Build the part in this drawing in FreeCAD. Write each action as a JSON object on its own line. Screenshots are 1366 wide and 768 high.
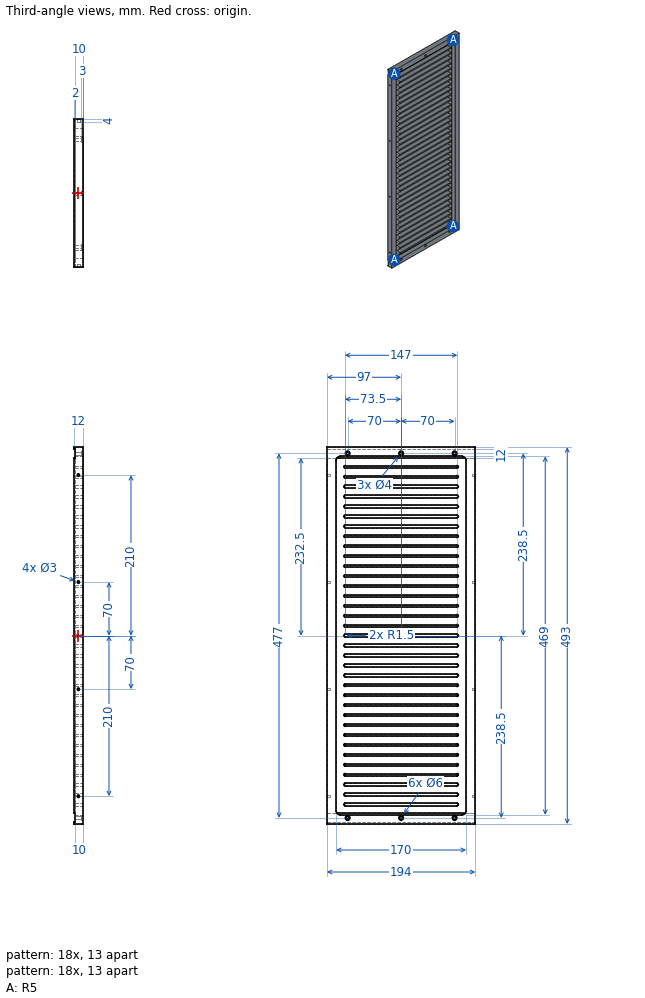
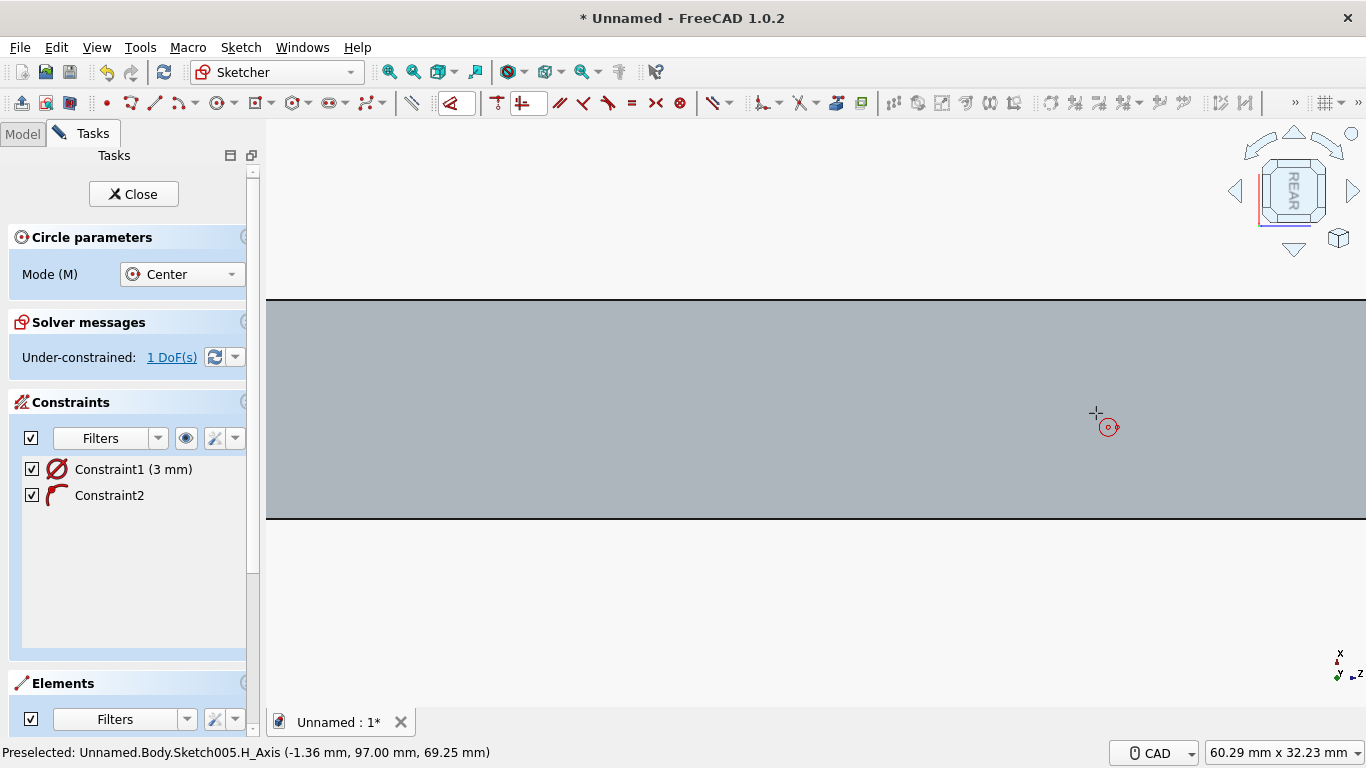
{"action": "scroll", "coordinate": [1096, 413], "scroll_direction": "down", "scroll_amount": 12}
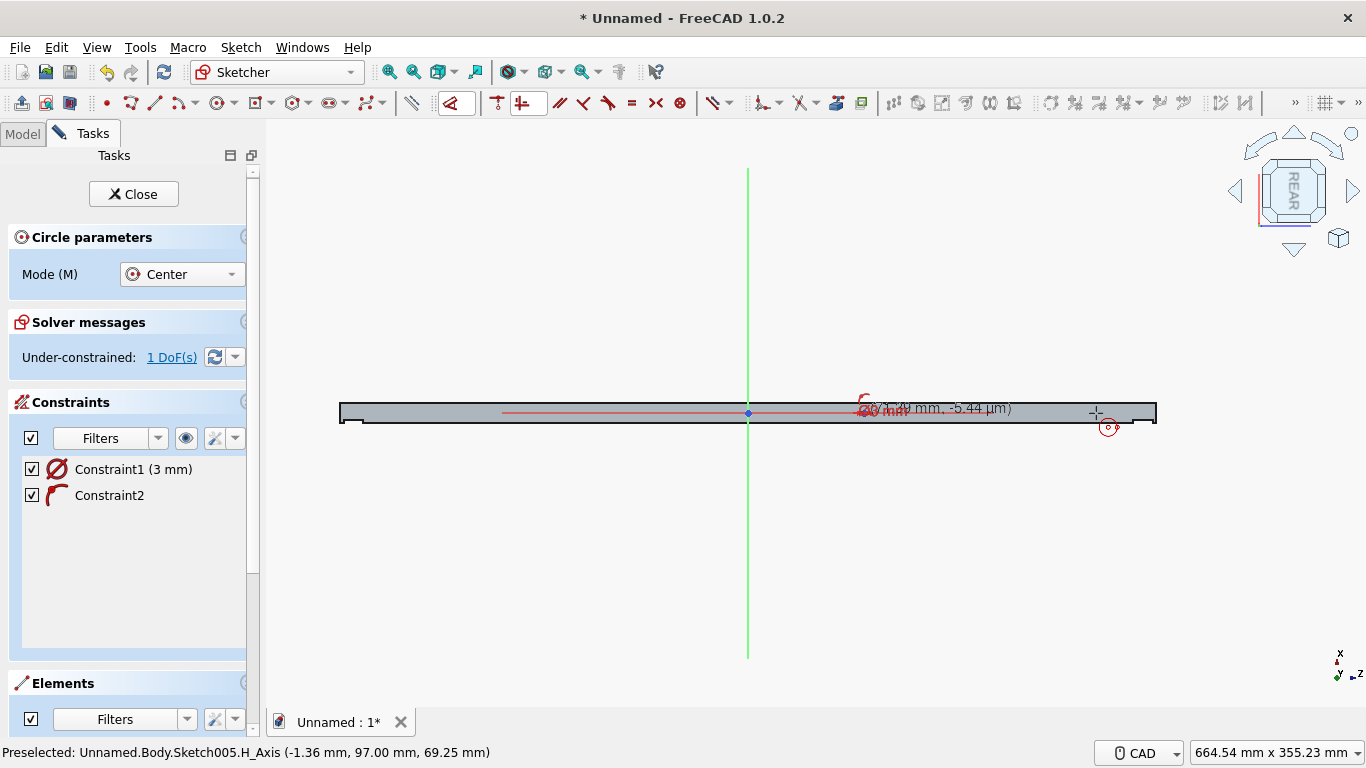
{"action": "left_click", "coordinate": [1096, 413]}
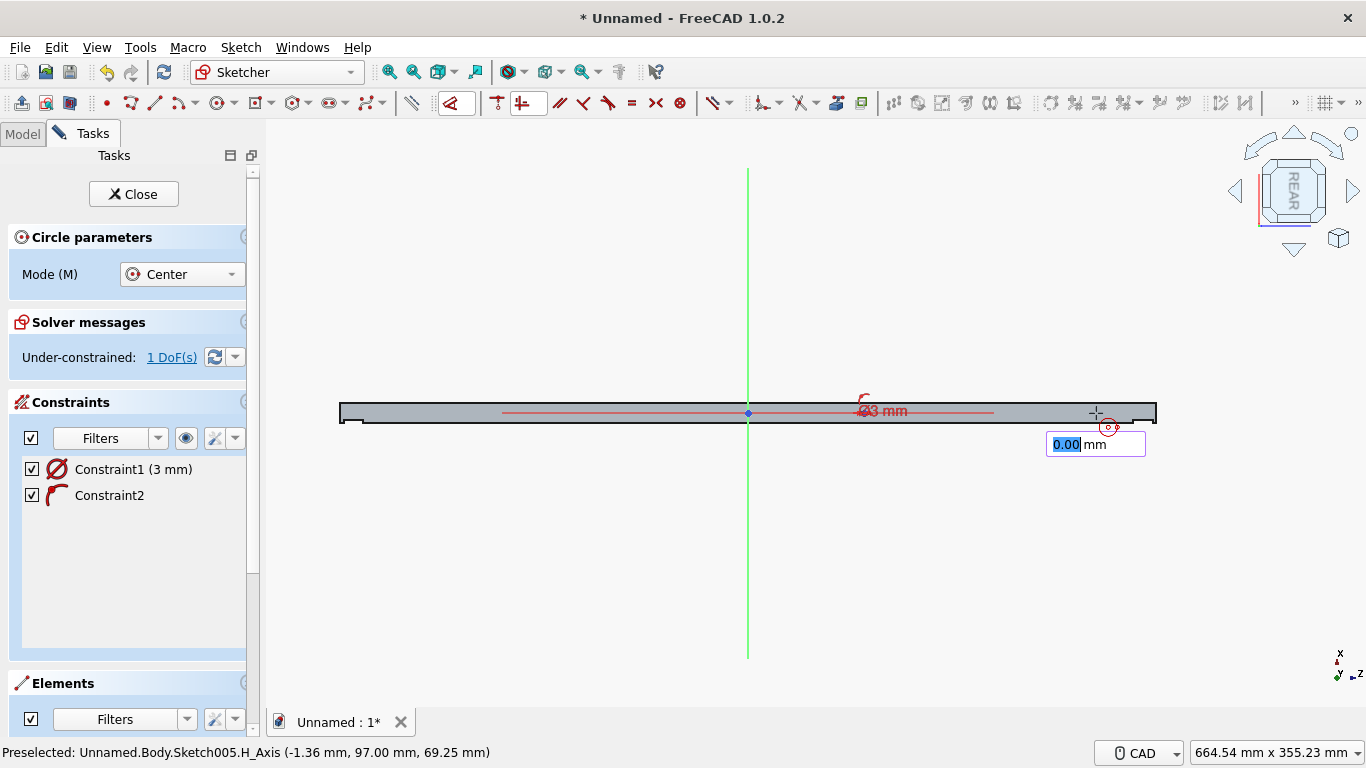
{"action": "scroll", "coordinate": [1095, 415], "scroll_direction": "up", "scroll_amount": 10}
{"action": "mouse_move", "coordinate": [1091, 415]}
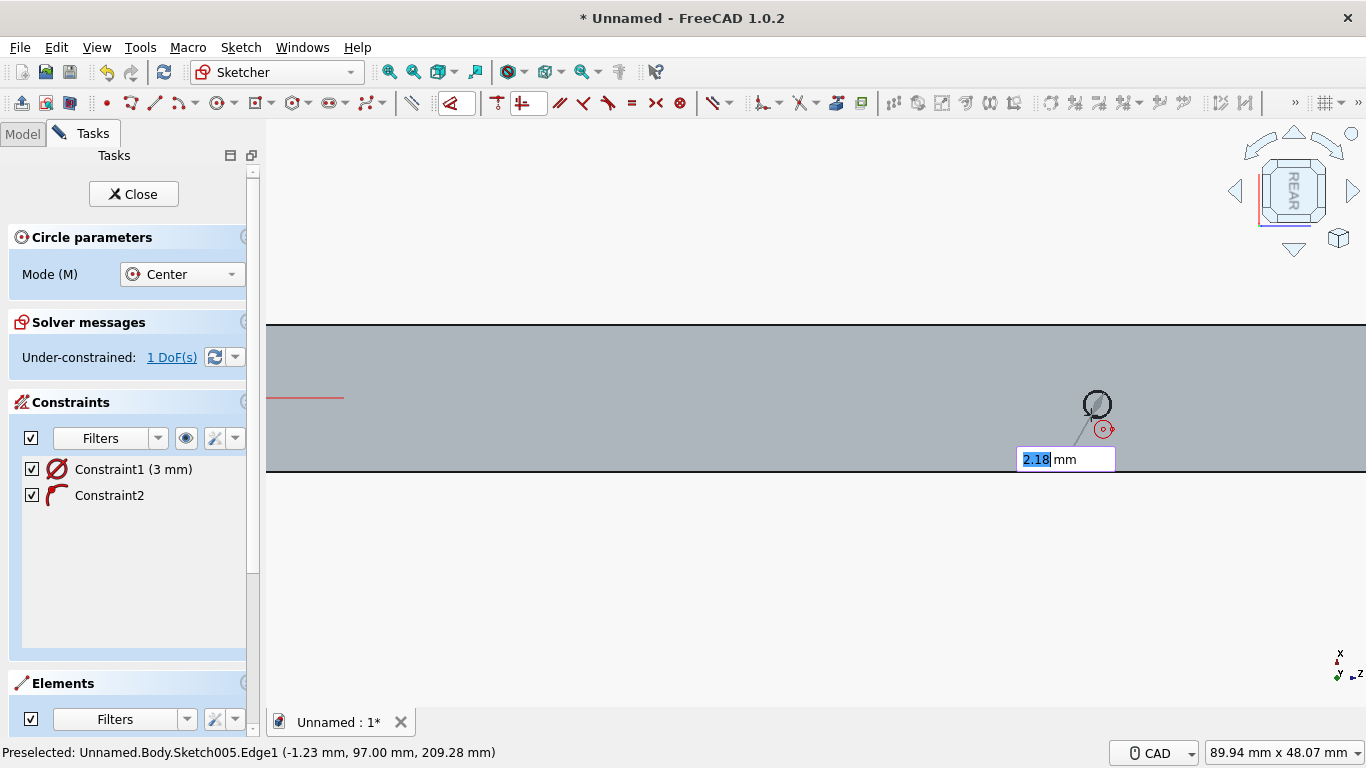
{"action": "type", "text": "3"}
{"action": "key", "text": "Return"}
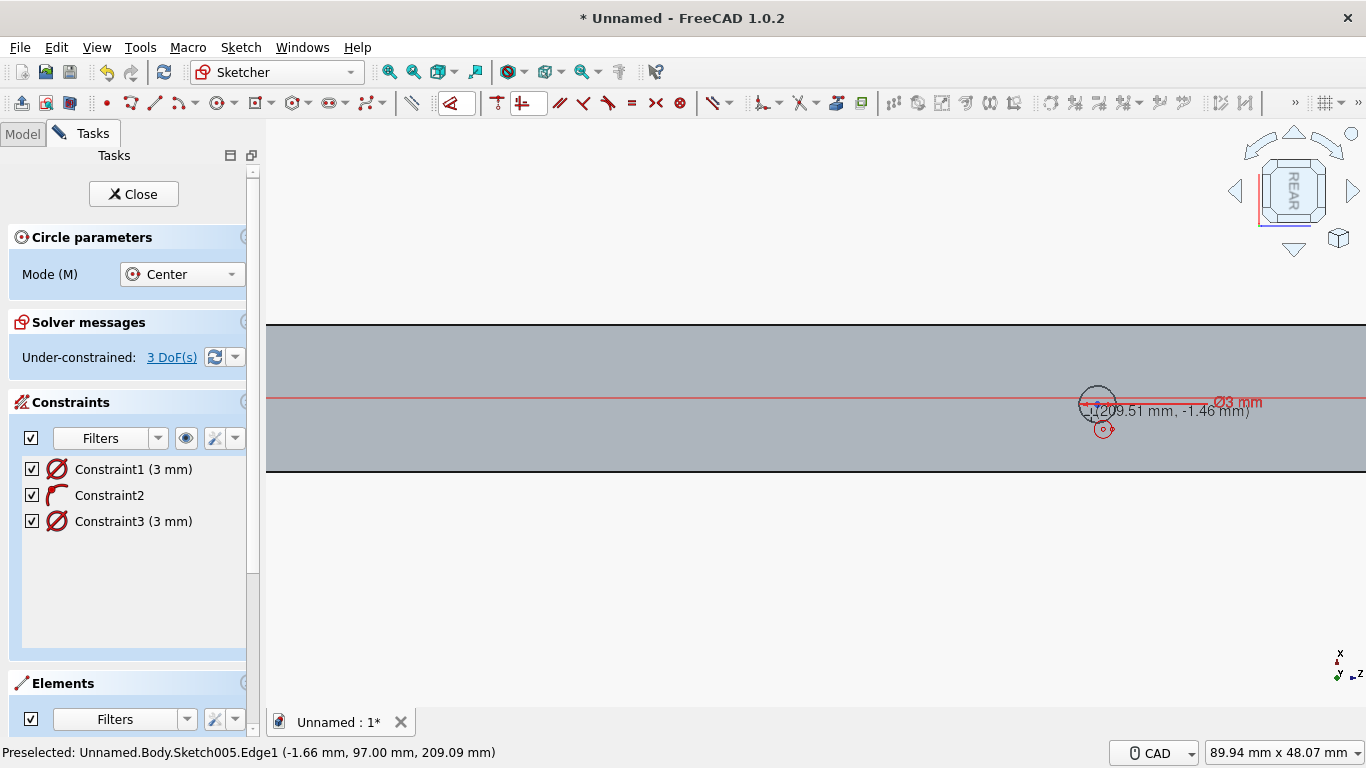
{"action": "scroll", "coordinate": [1095, 415], "scroll_direction": "down", "scroll_amount": 10}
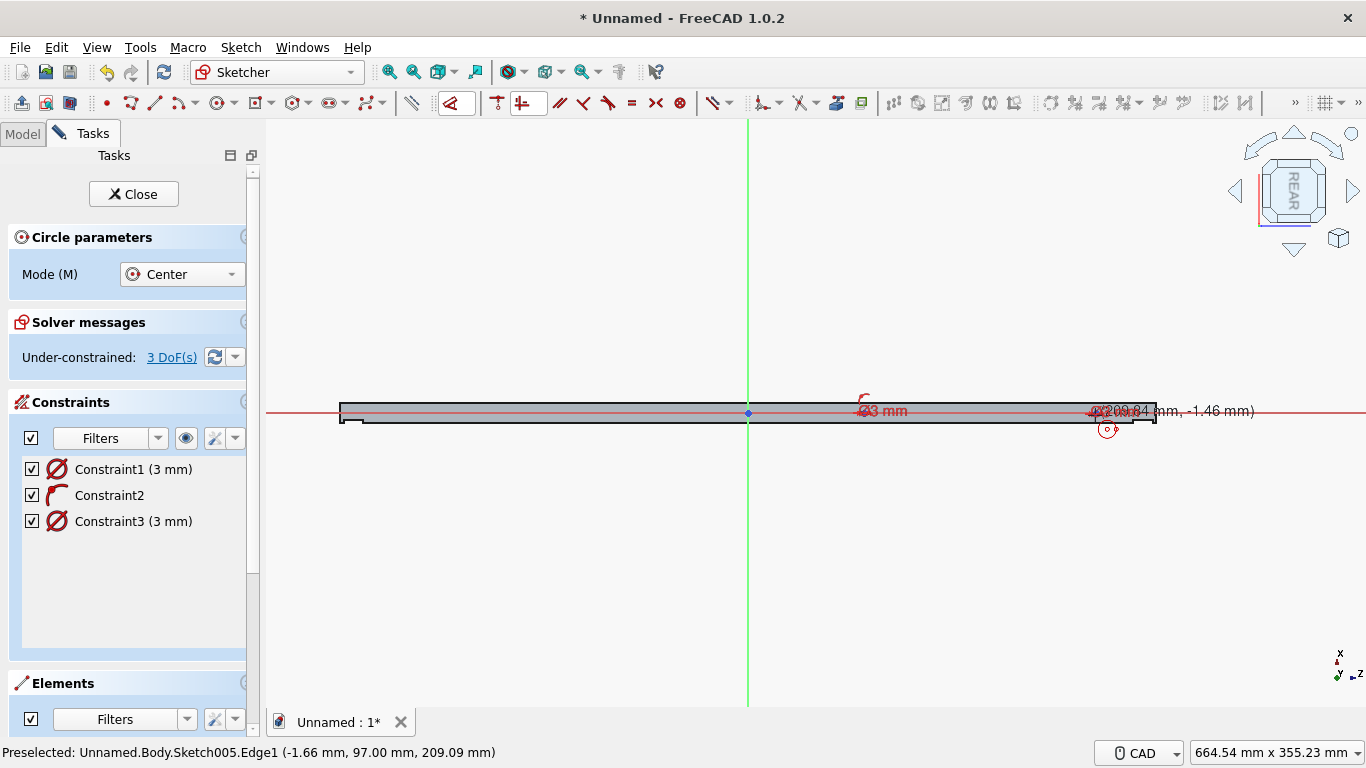
{"action": "scroll", "coordinate": [401, 413], "scroll_direction": "up", "scroll_amount": 12}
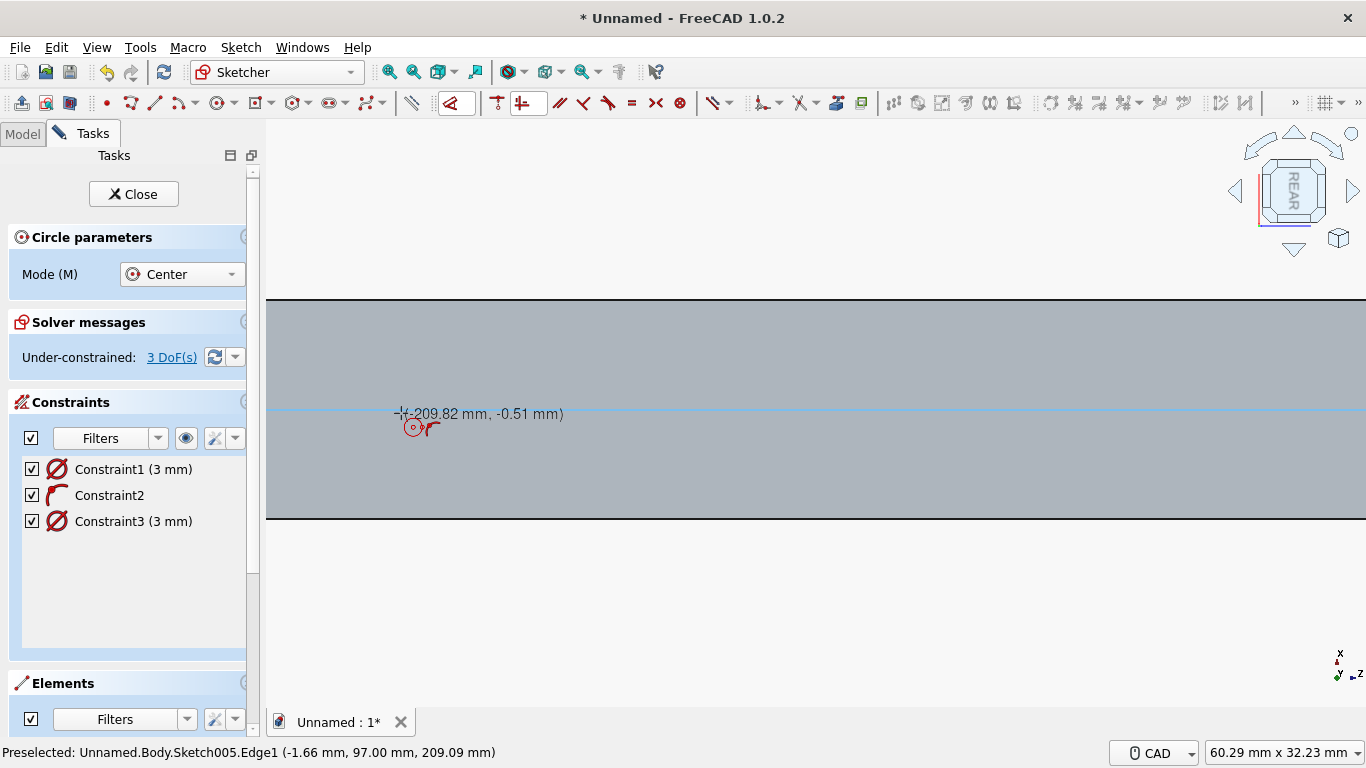
{"action": "scroll", "coordinate": [400, 413], "scroll_direction": "down", "scroll_amount": 12}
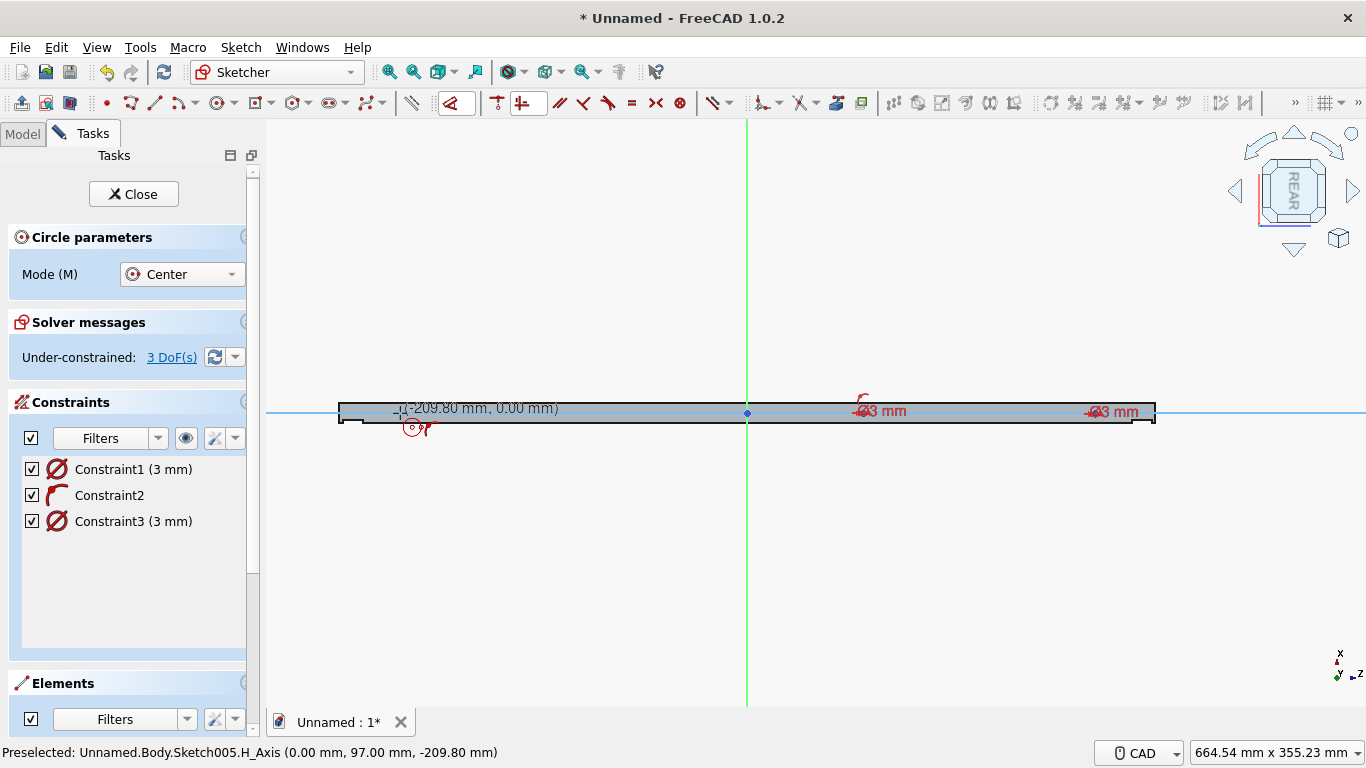
{"action": "left_click", "coordinate": [400, 413]}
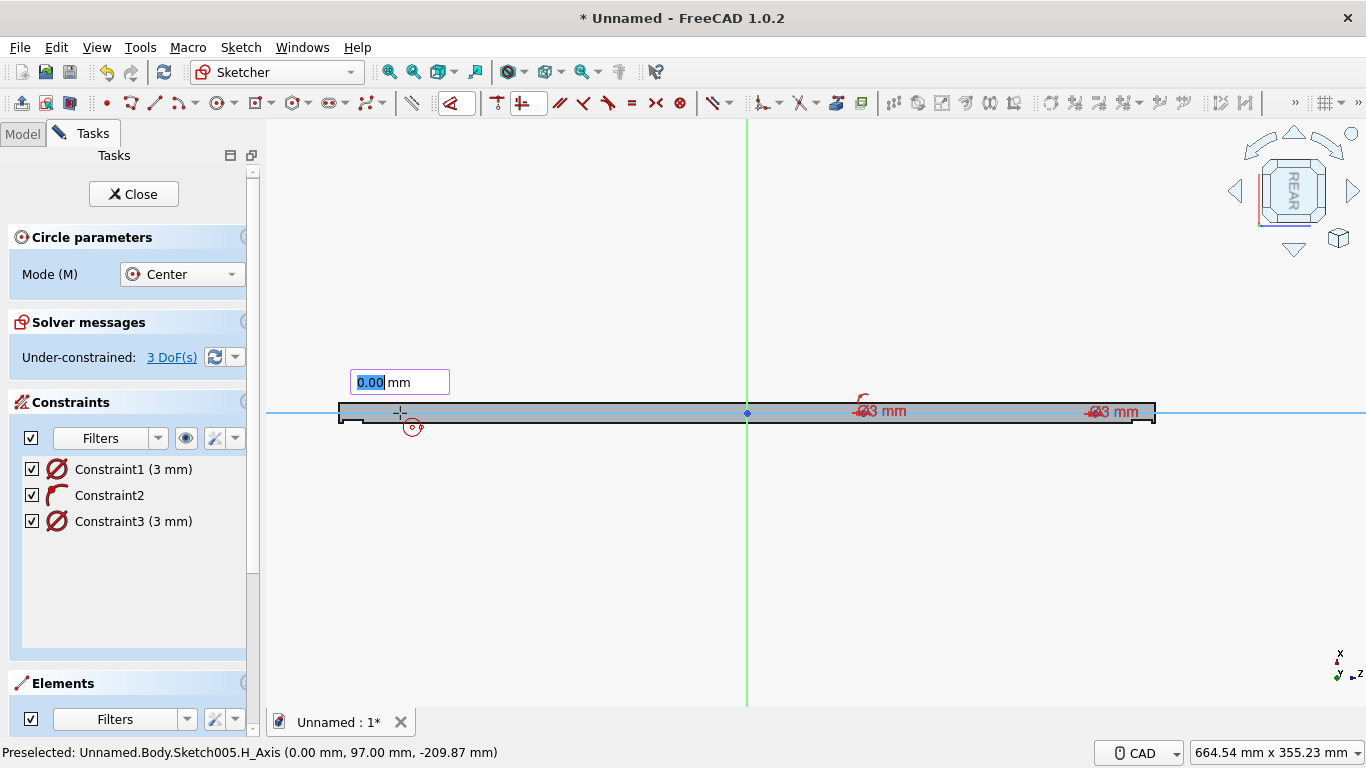
{"action": "scroll", "coordinate": [399, 415], "scroll_direction": "up", "scroll_amount": 10}
{"action": "mouse_move", "coordinate": [398, 415]}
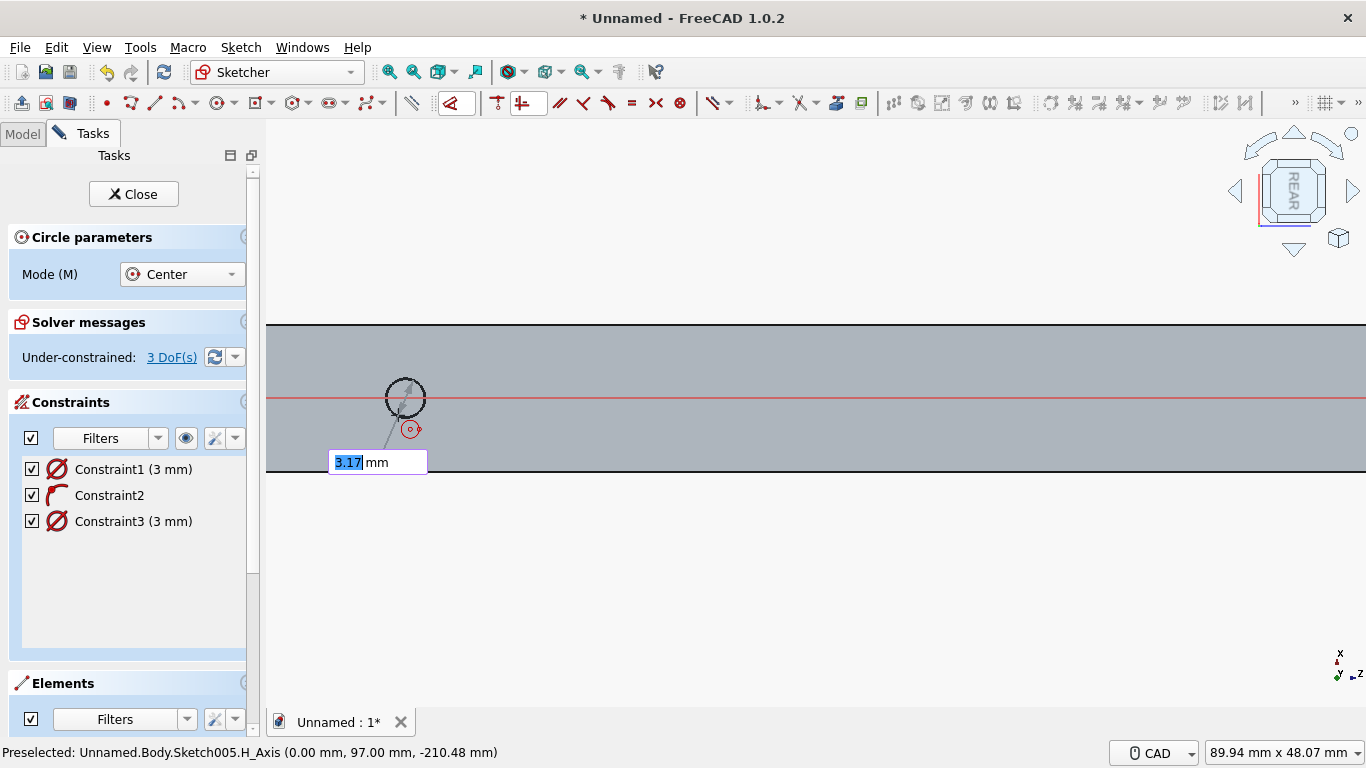
{"action": "type", "text": "3"}
{"action": "key", "text": "Return"}